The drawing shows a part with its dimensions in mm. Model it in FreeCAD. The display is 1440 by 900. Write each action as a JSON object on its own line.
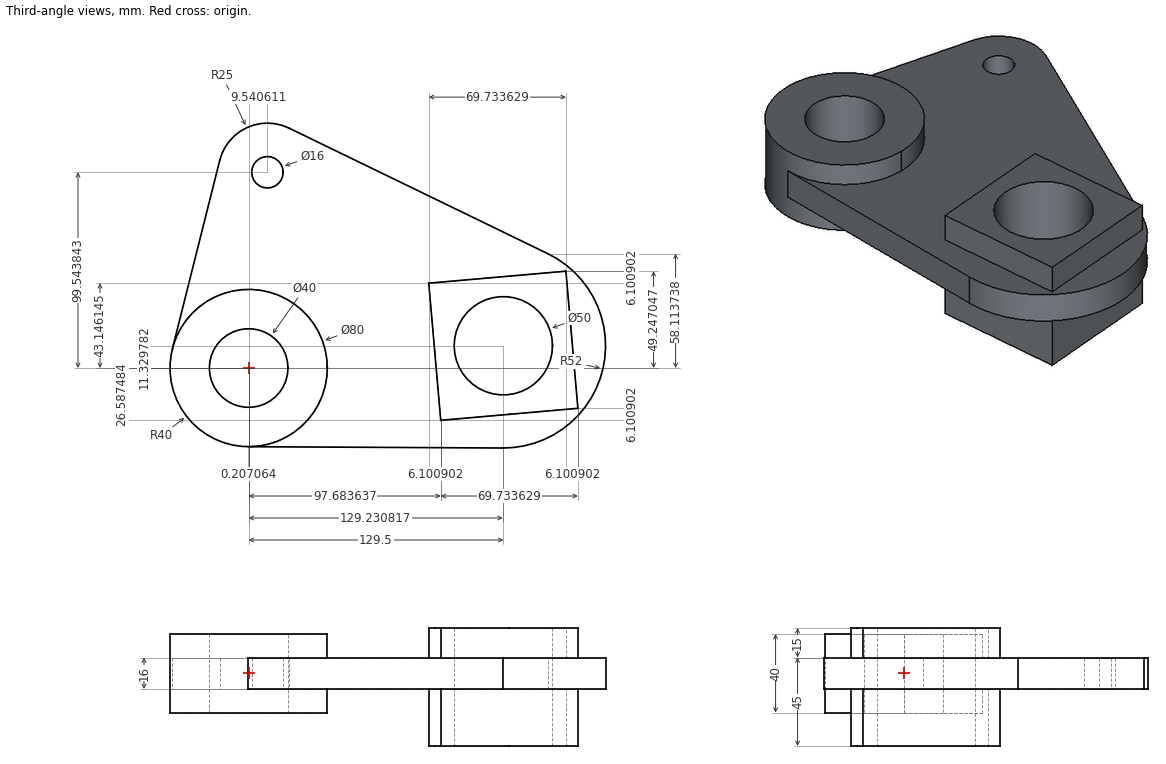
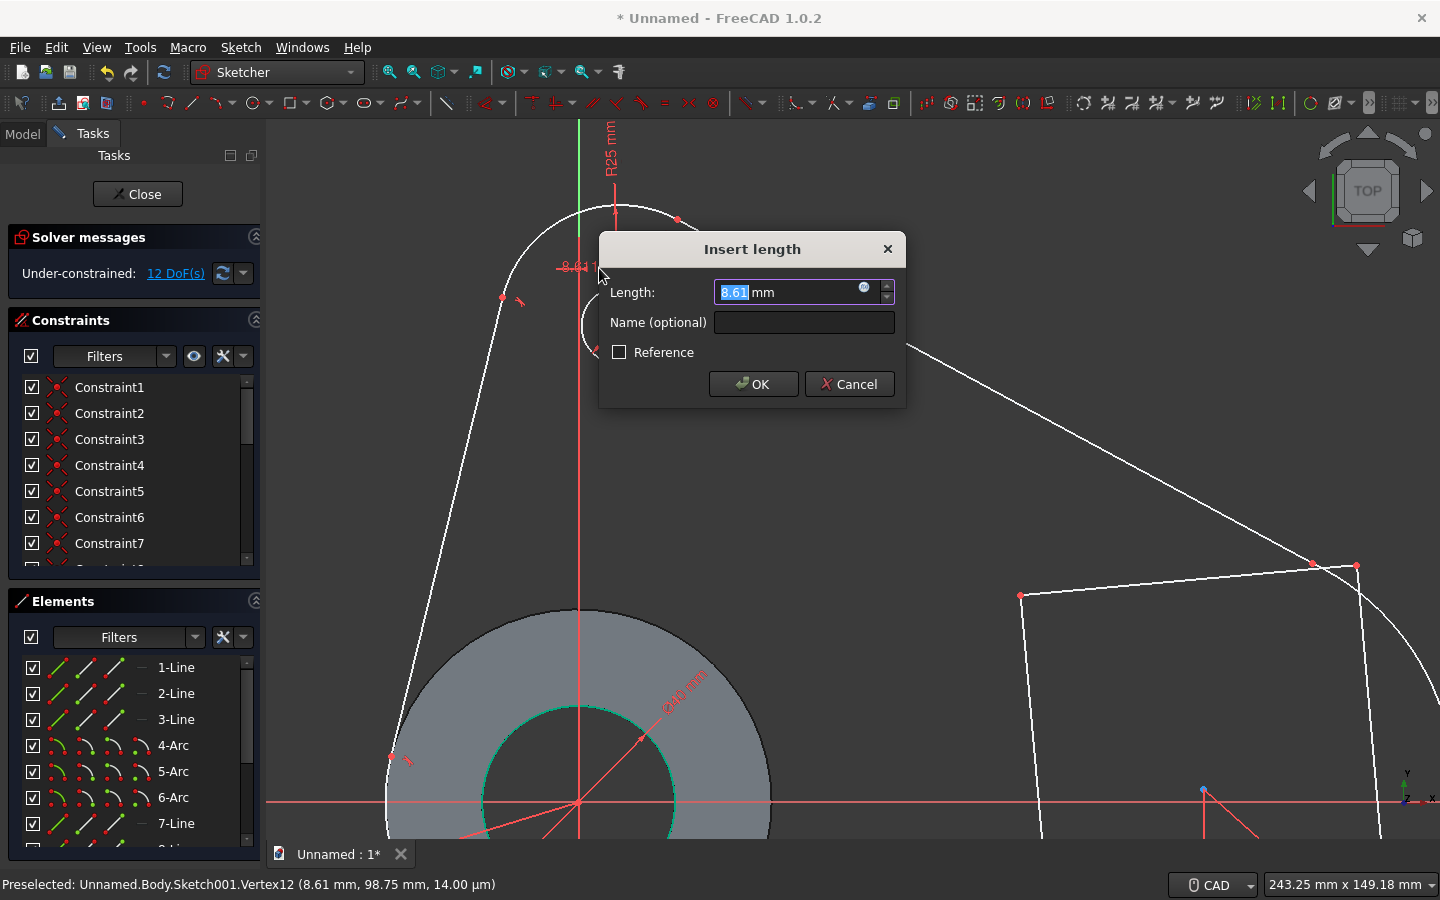
{"action": "type", "text": "9.540611"}
{"action": "key", "text": "Return"}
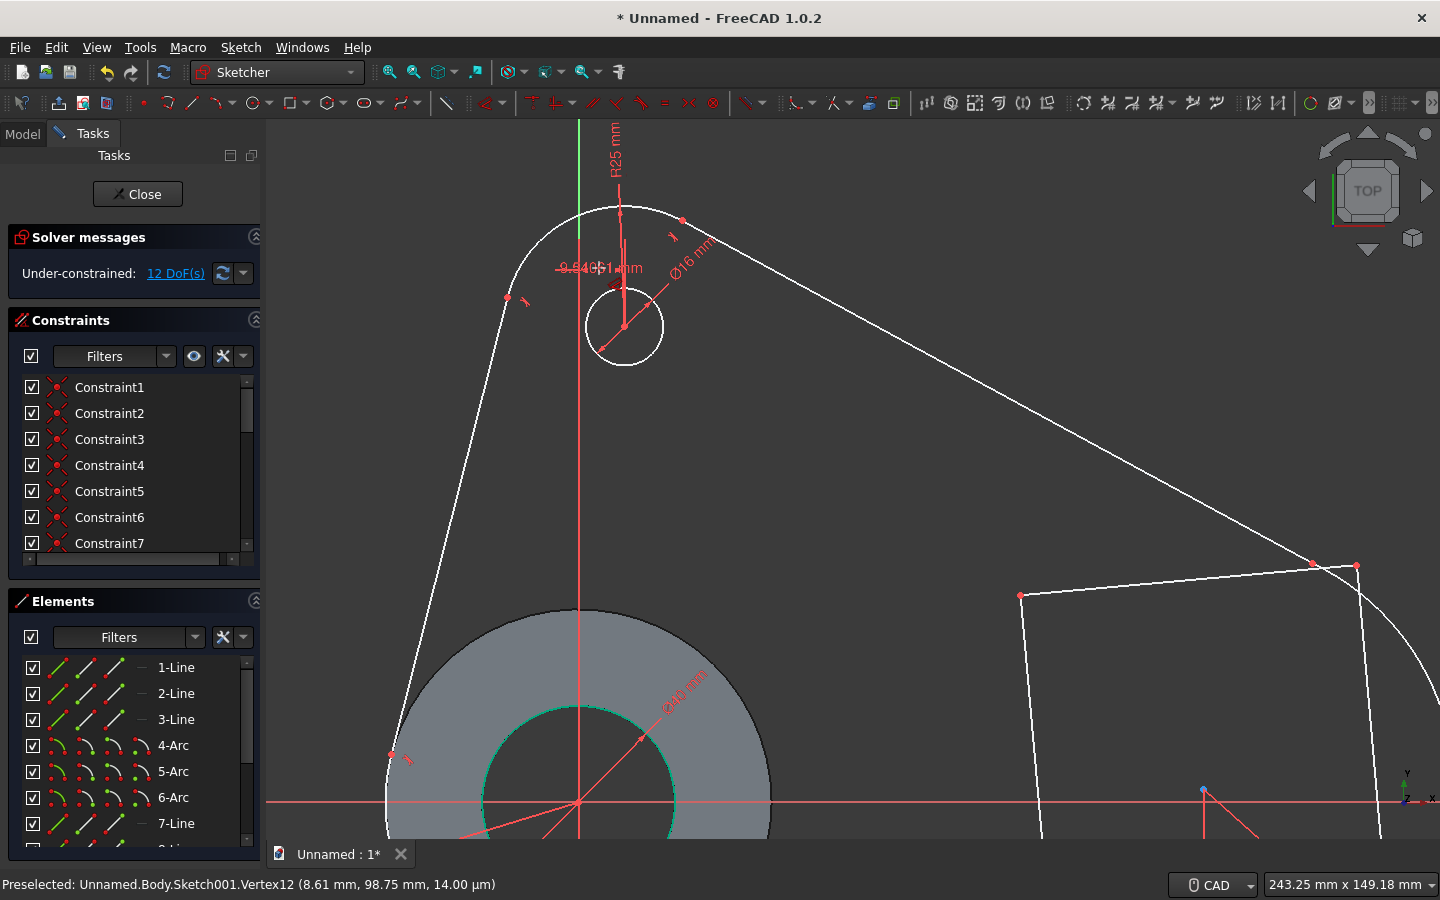
{"action": "scroll", "coordinate": [620, 325], "scroll_direction": "down", "scroll_amount": 3}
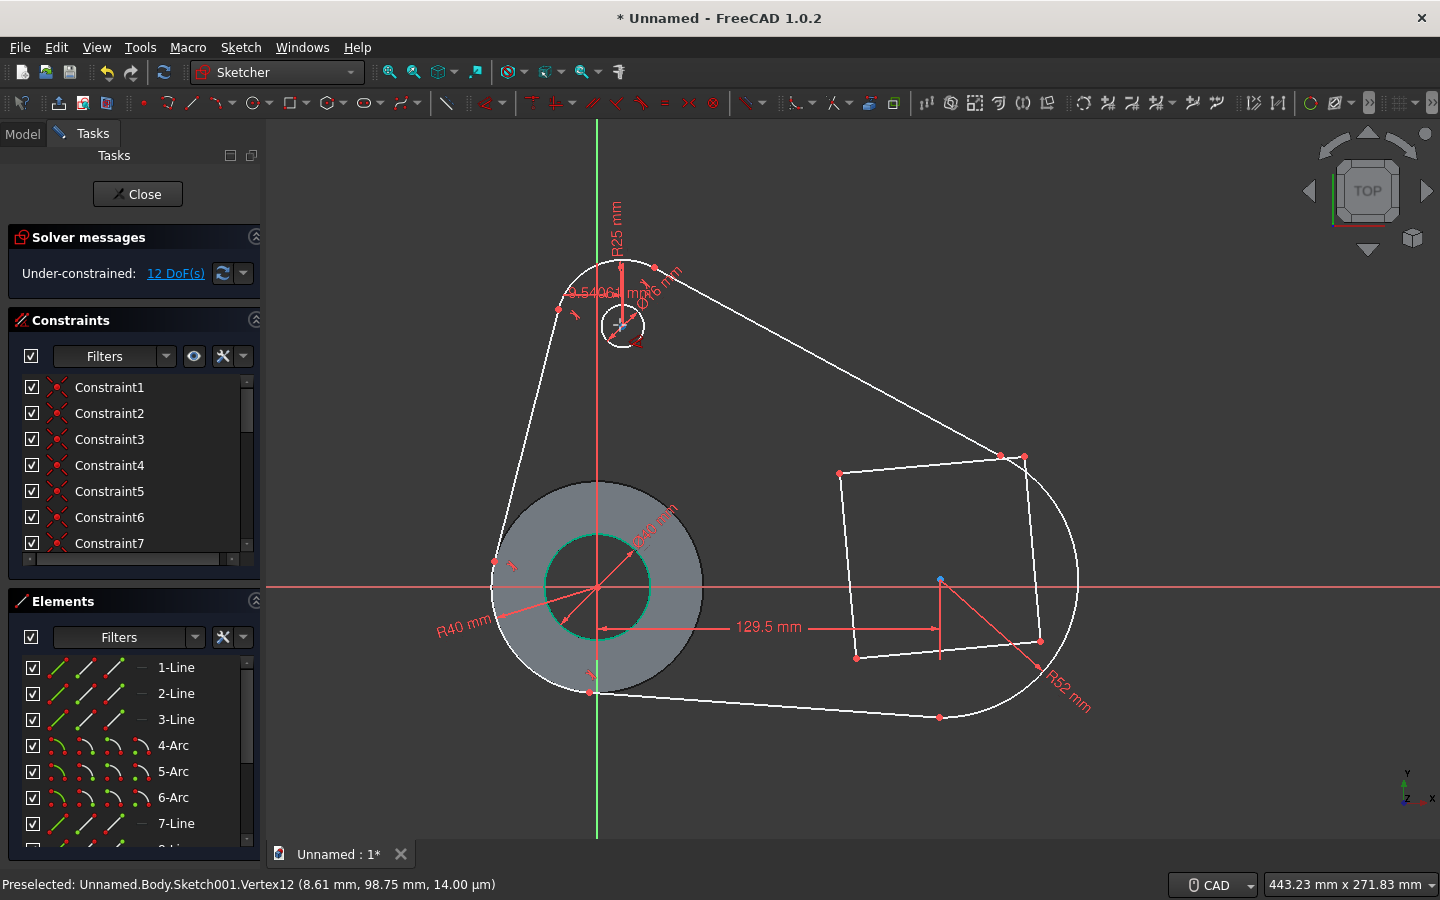
{"action": "scroll", "coordinate": [590, 693], "scroll_direction": "up", "scroll_amount": 22}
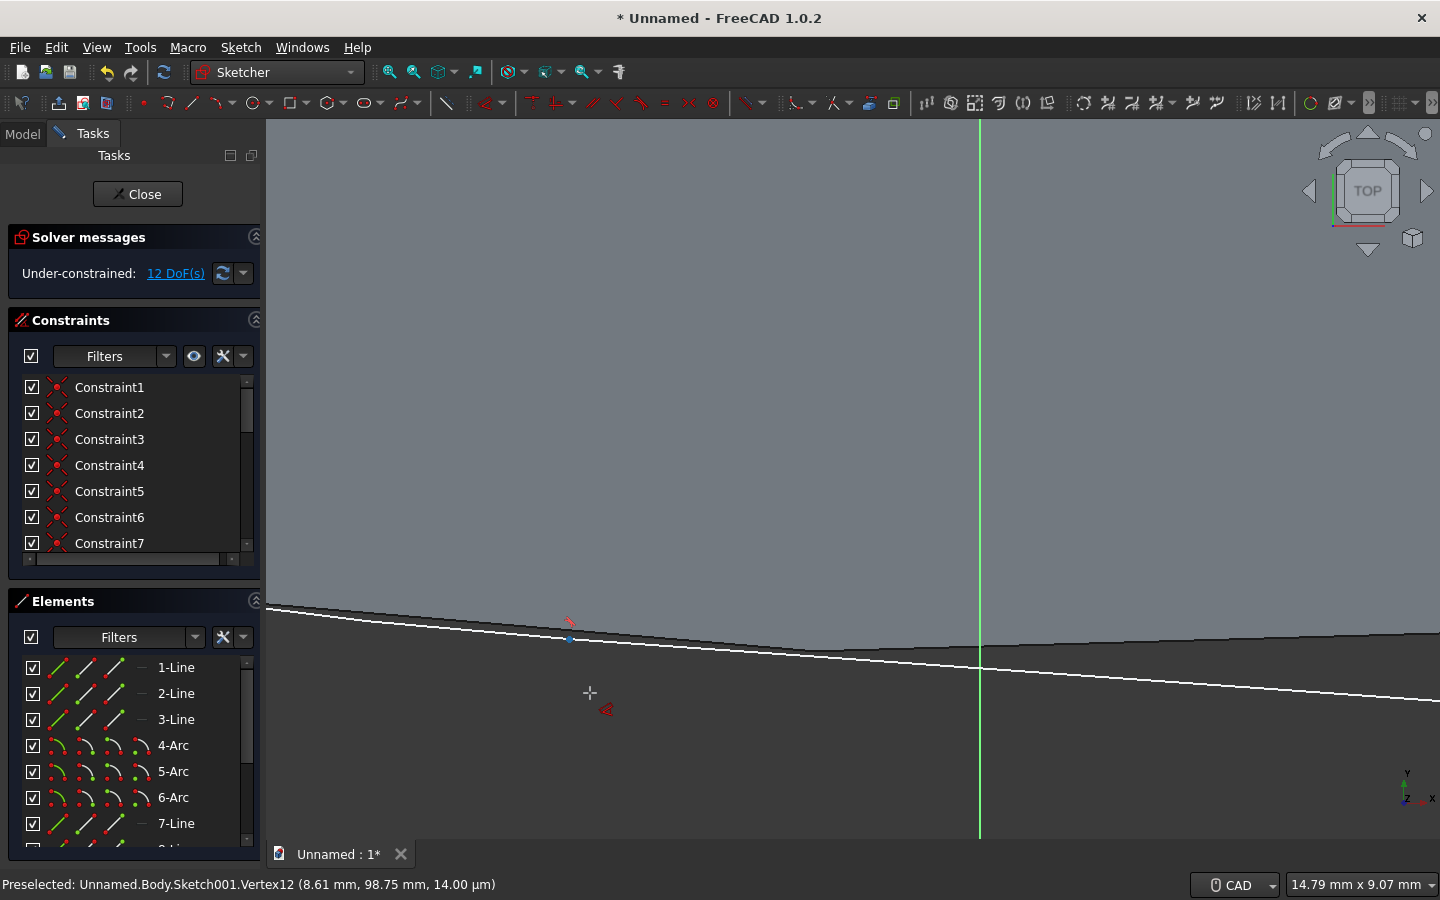
{"action": "left_click", "coordinate": [559, 612]}
{"action": "left_click", "coordinate": [724, 646]}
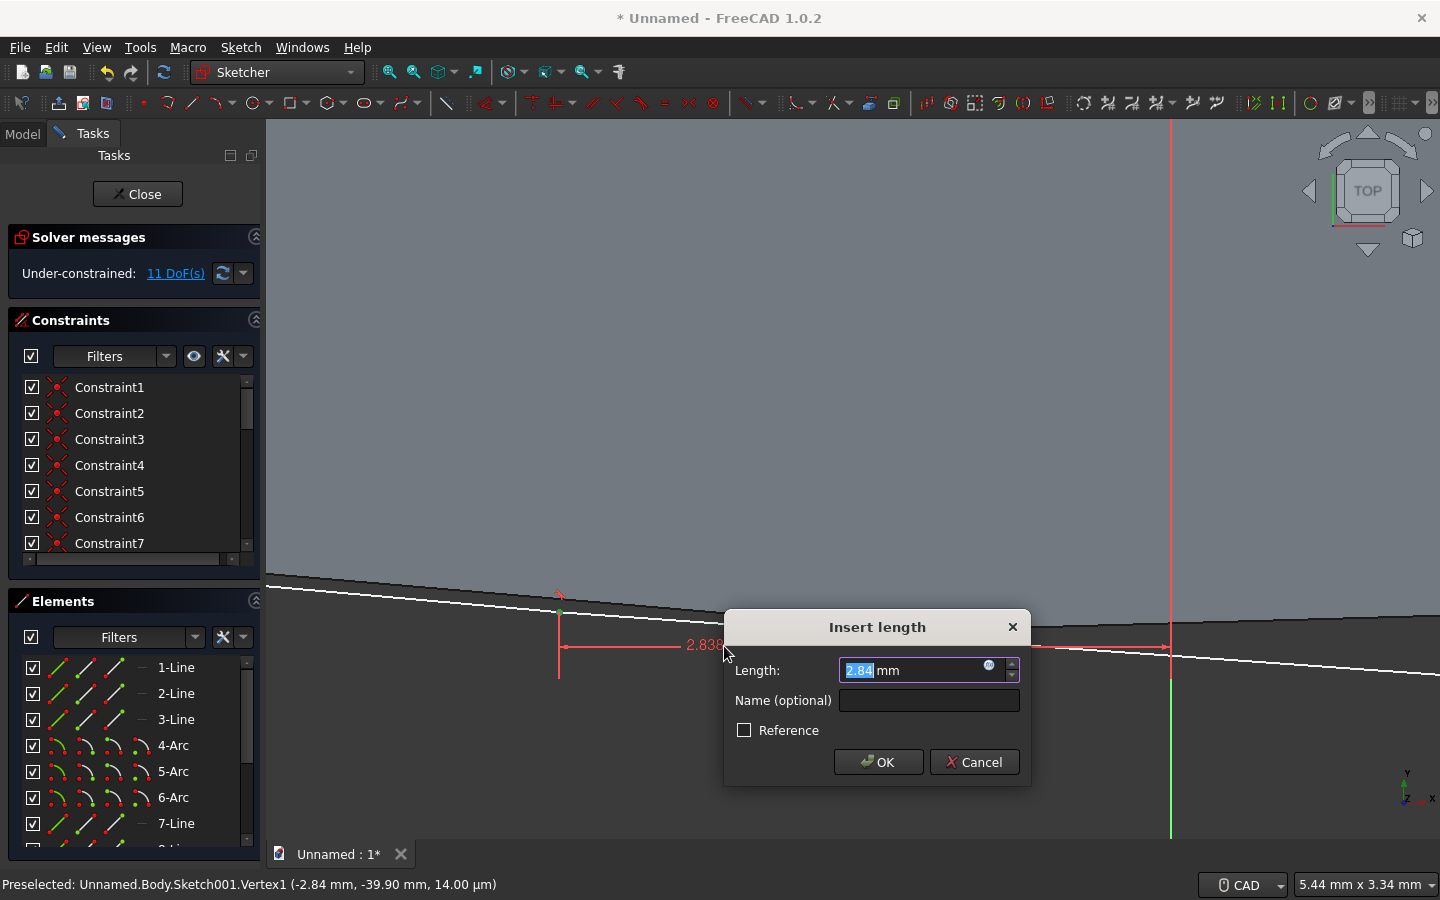
{"action": "type", "text": "0.207064"}
{"action": "key", "text": "Return"}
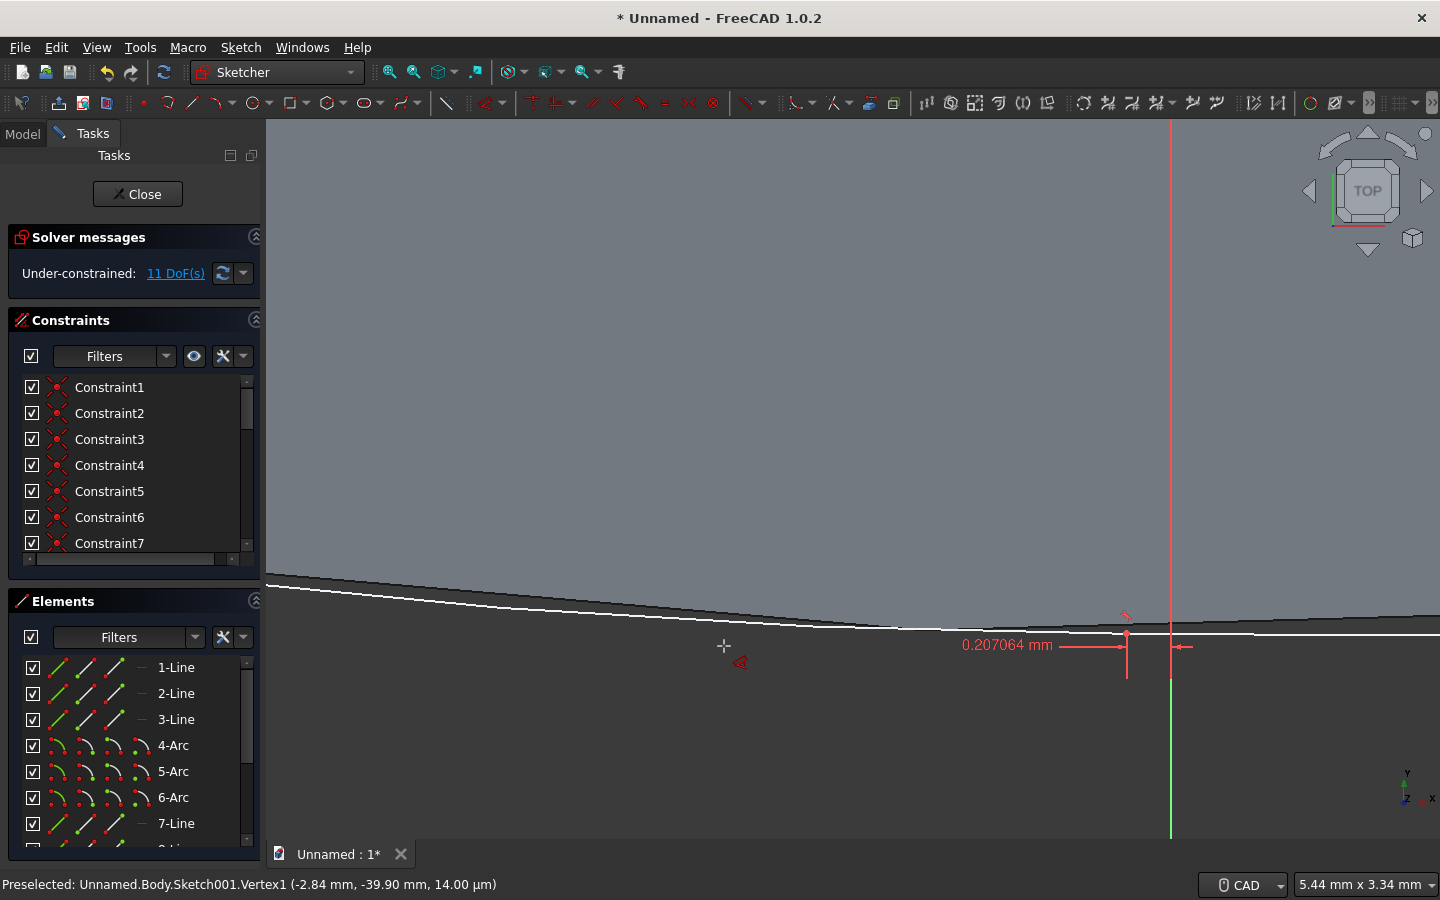
{"action": "scroll", "coordinate": [784, 479], "scroll_direction": "down", "scroll_amount": 15}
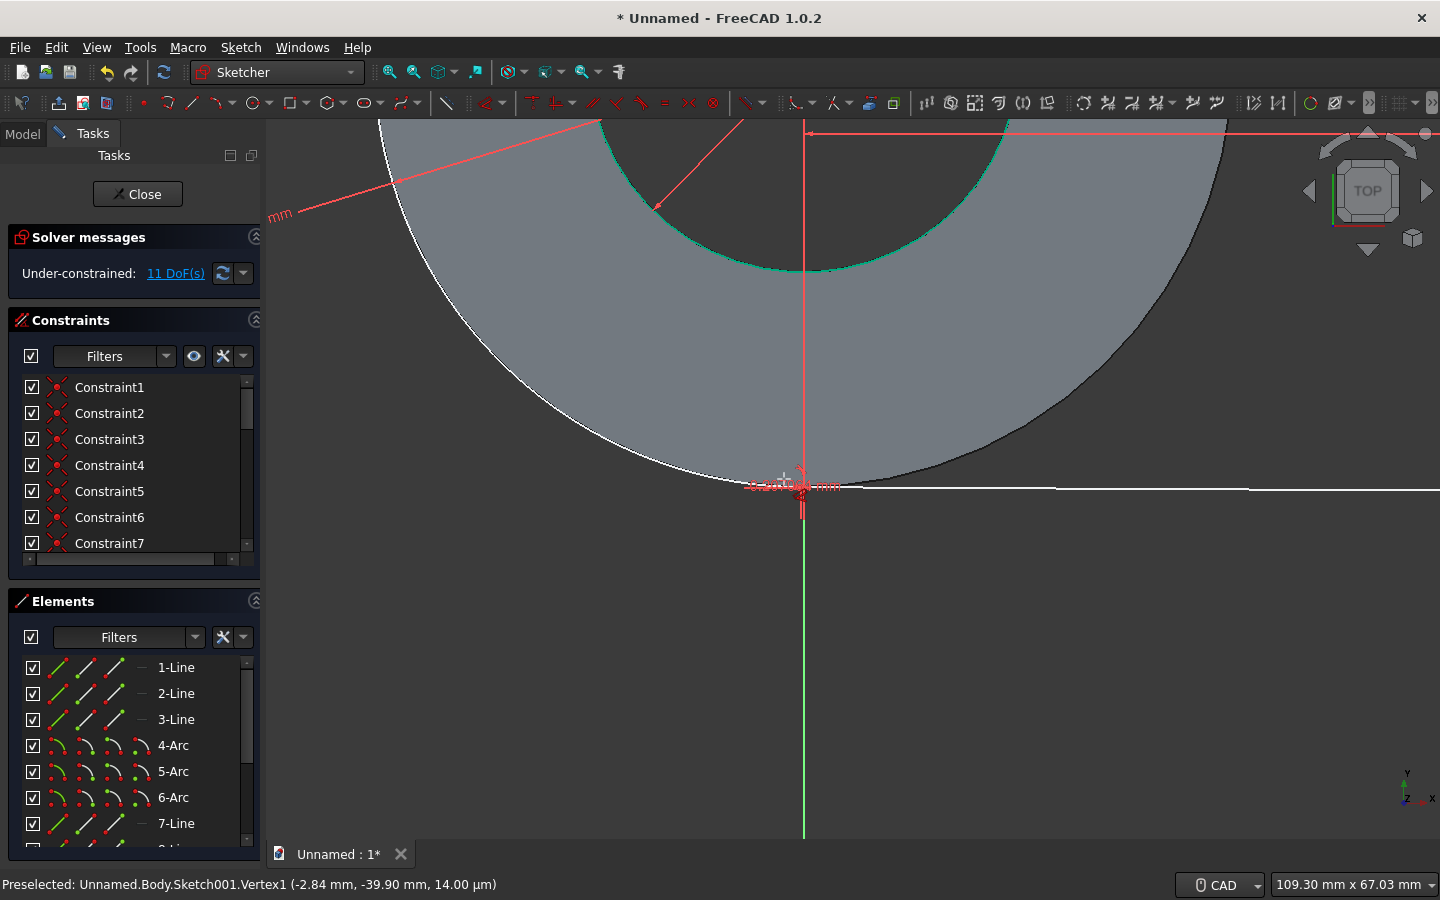
{"action": "scroll", "coordinate": [530, 760], "scroll_direction": "down", "scroll_amount": 7}